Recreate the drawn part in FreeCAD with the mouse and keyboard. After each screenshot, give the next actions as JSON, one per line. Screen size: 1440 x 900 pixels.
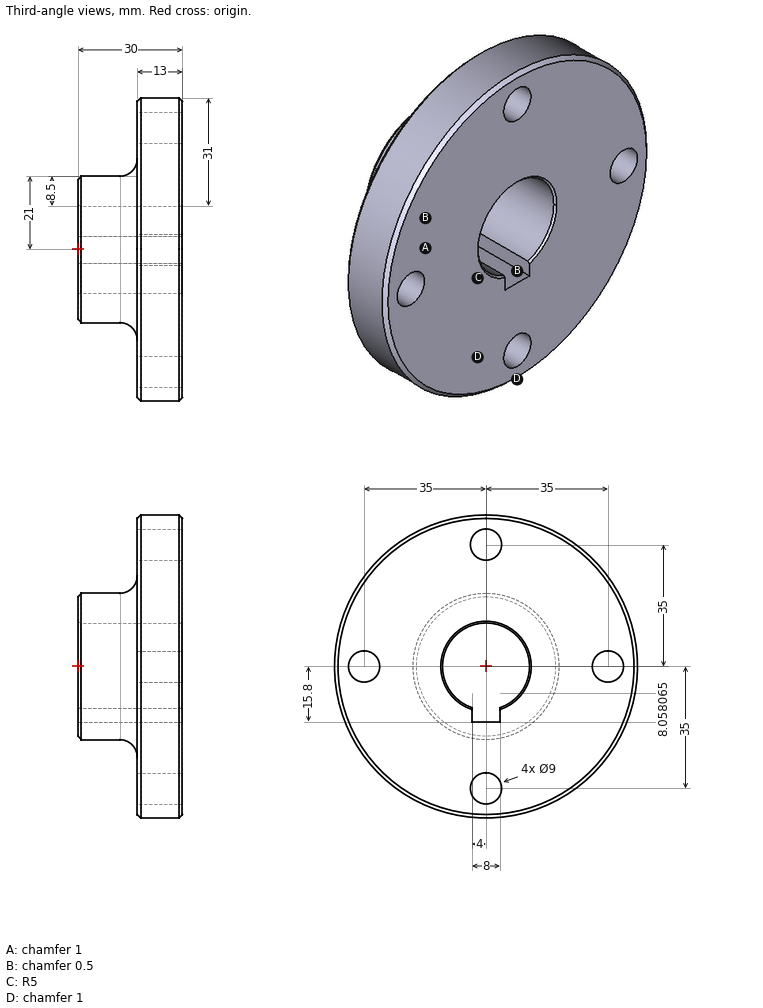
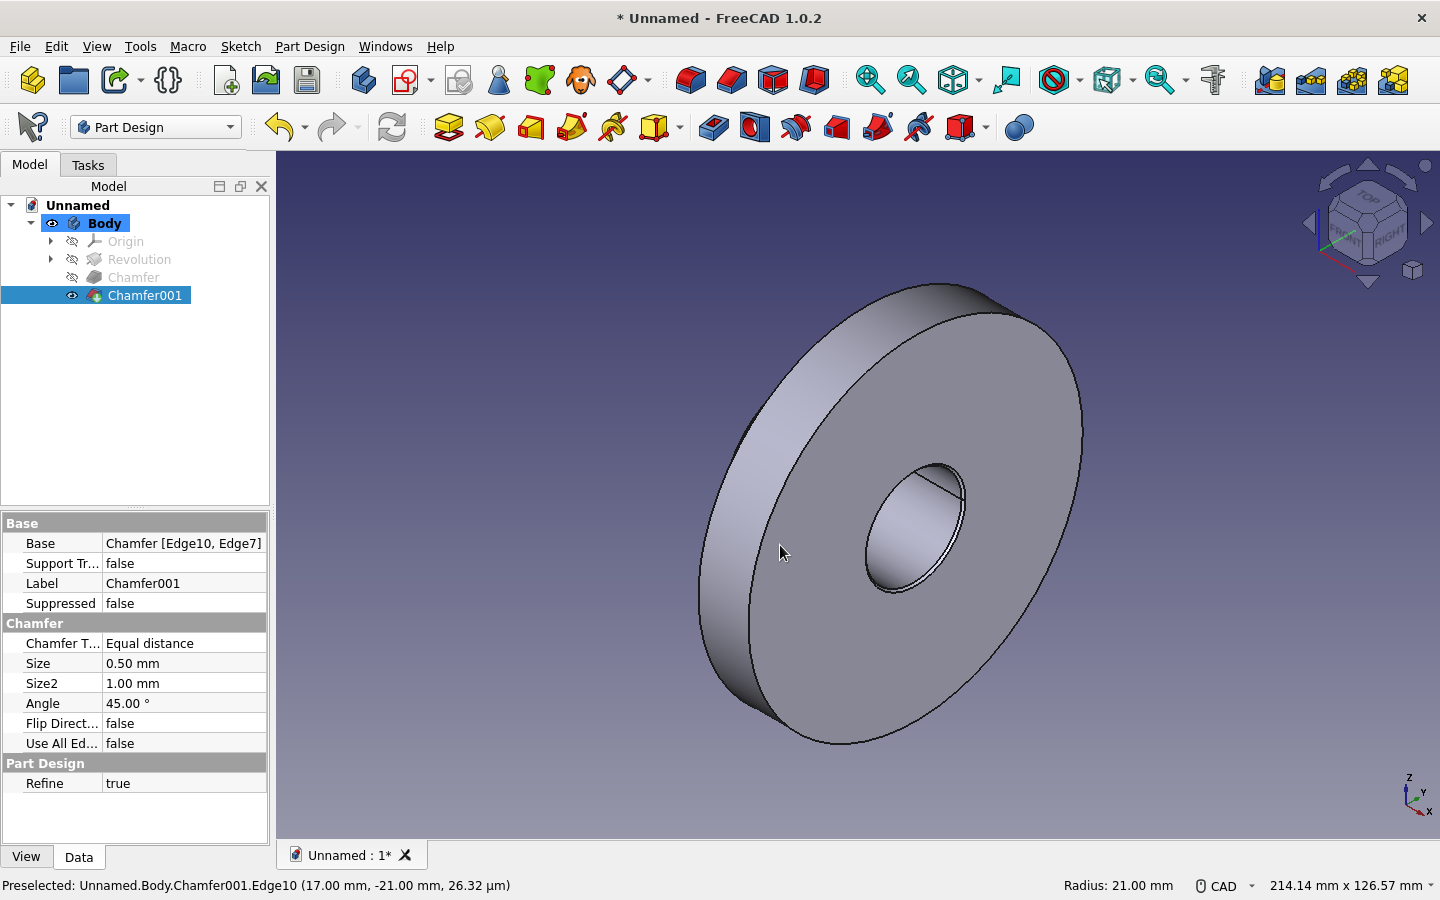
{"action": "left_click", "coordinate": [691, 80]}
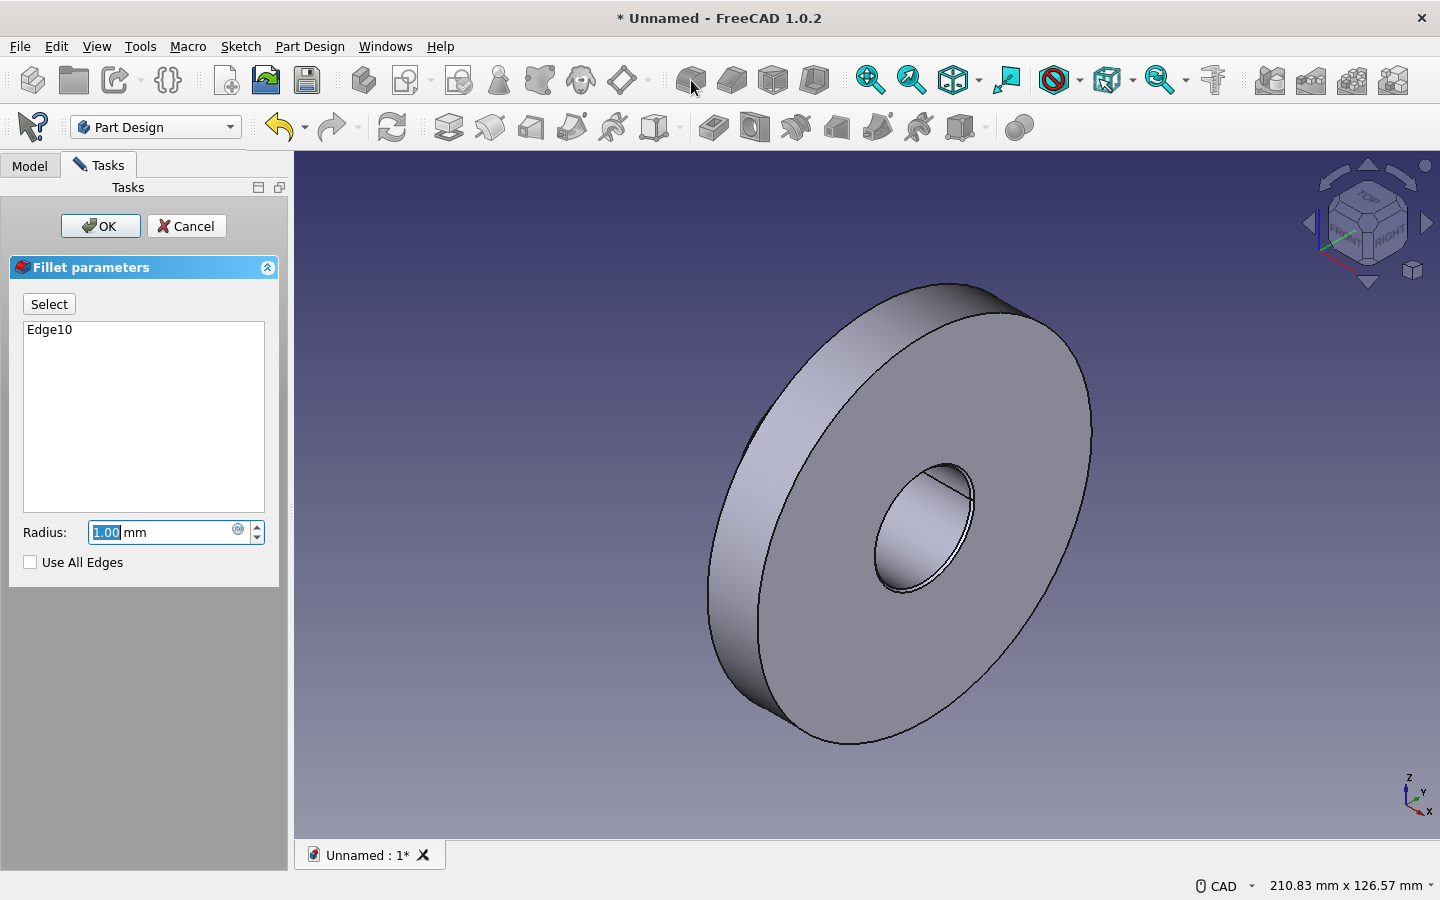
{"action": "type", "text": "5"}
{"action": "key", "text": "Tab"}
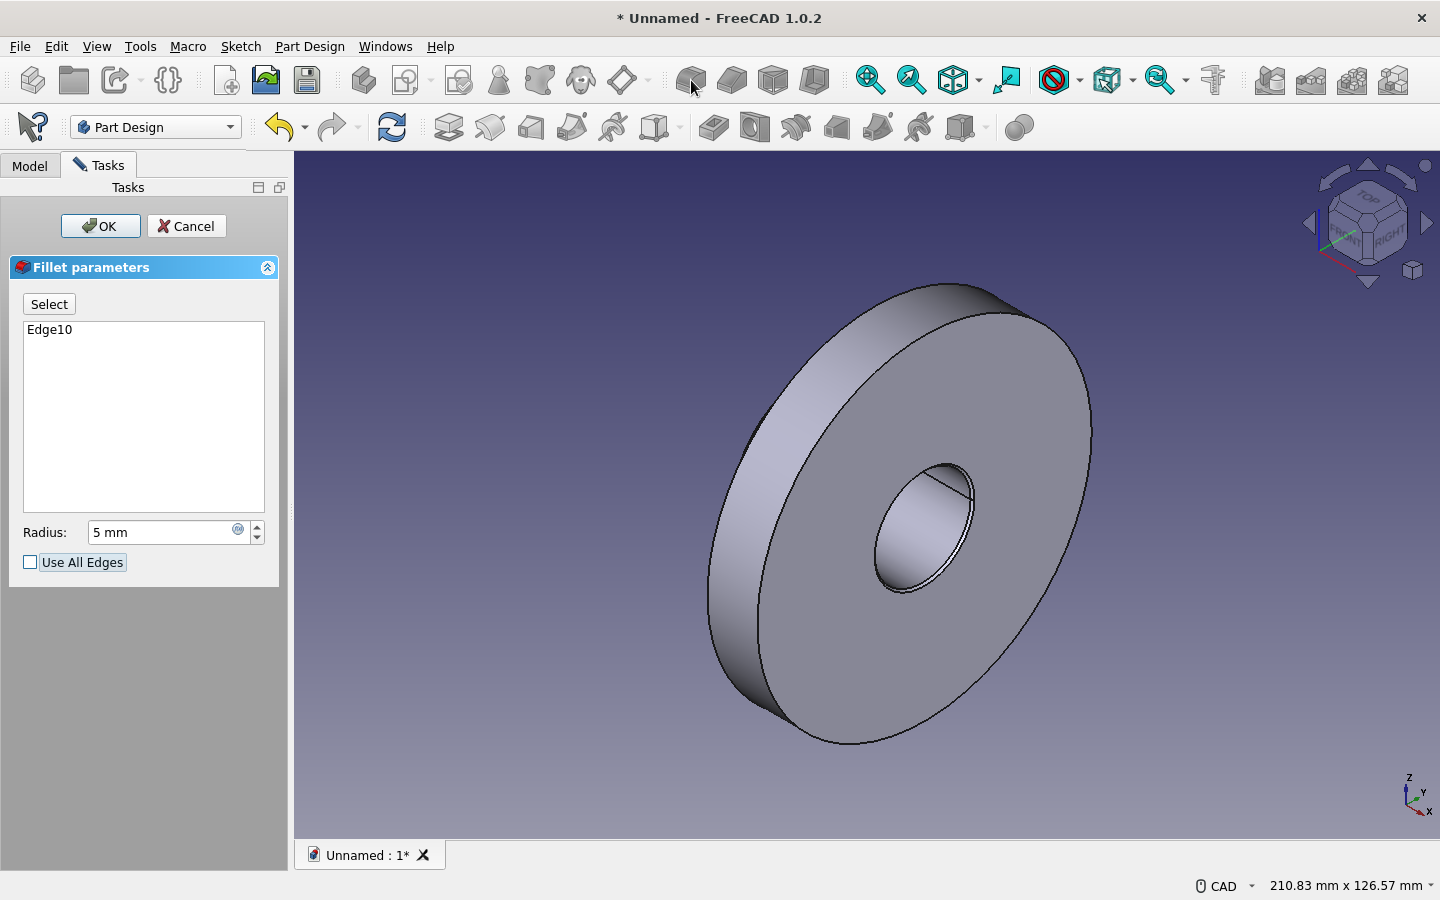
{"action": "left_click", "coordinate": [101, 226]}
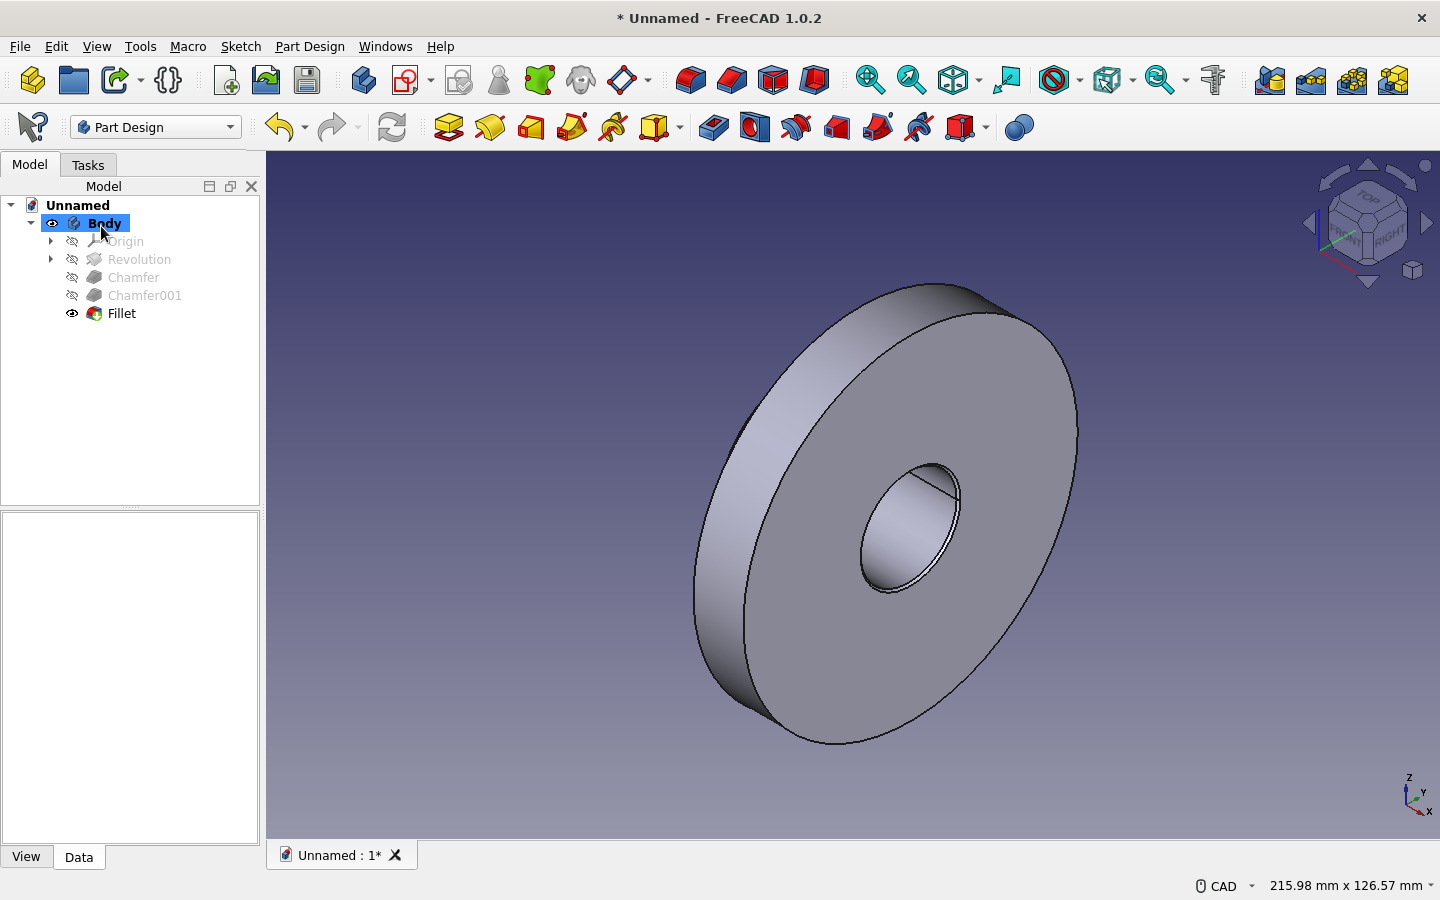
{"action": "left_click", "coordinate": [743, 624]}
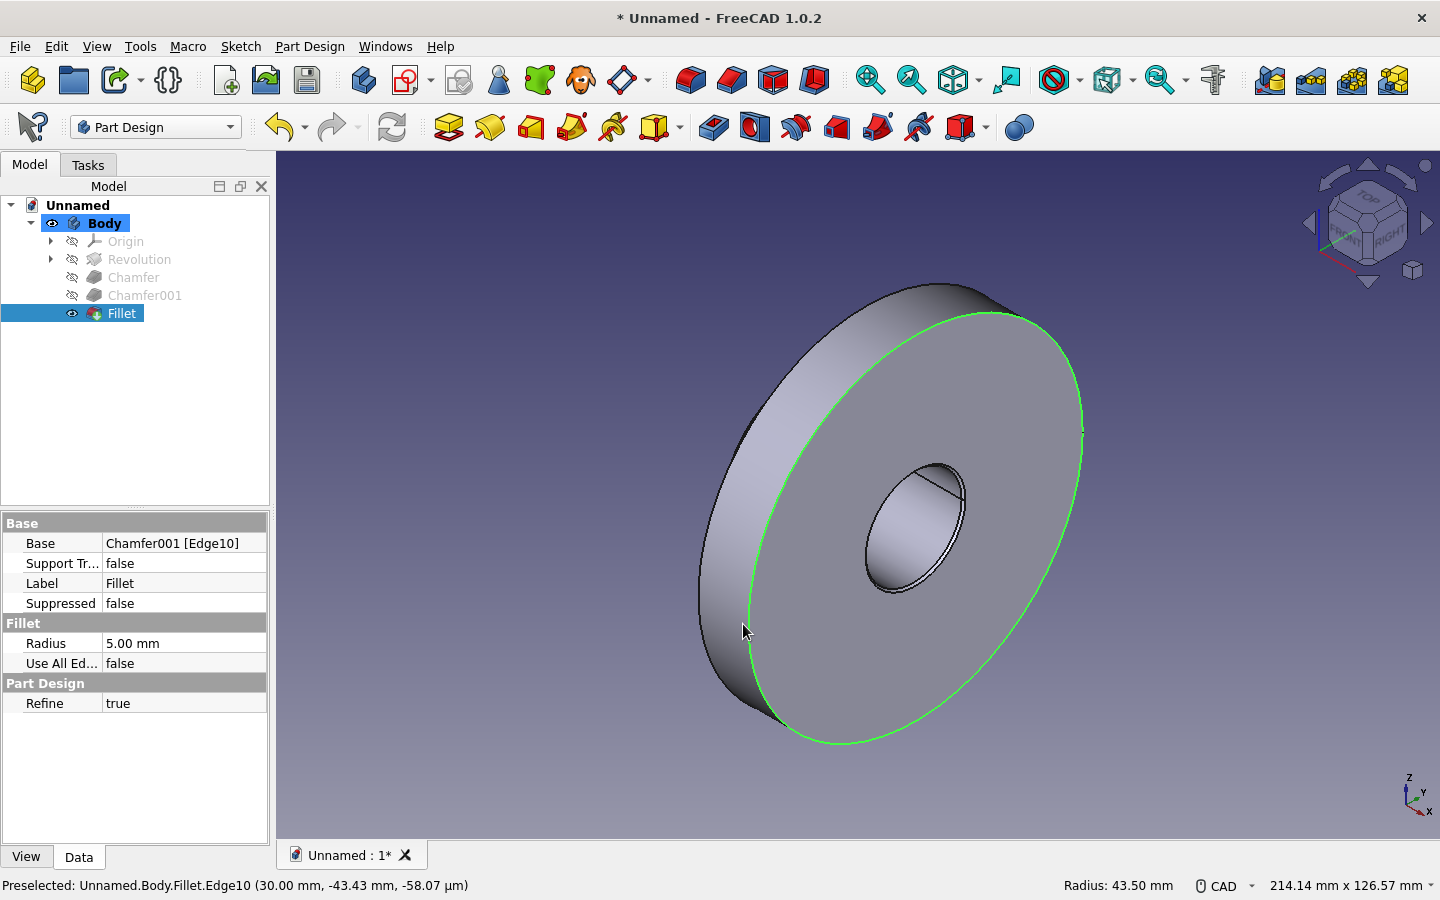
{"action": "key", "text": "2"}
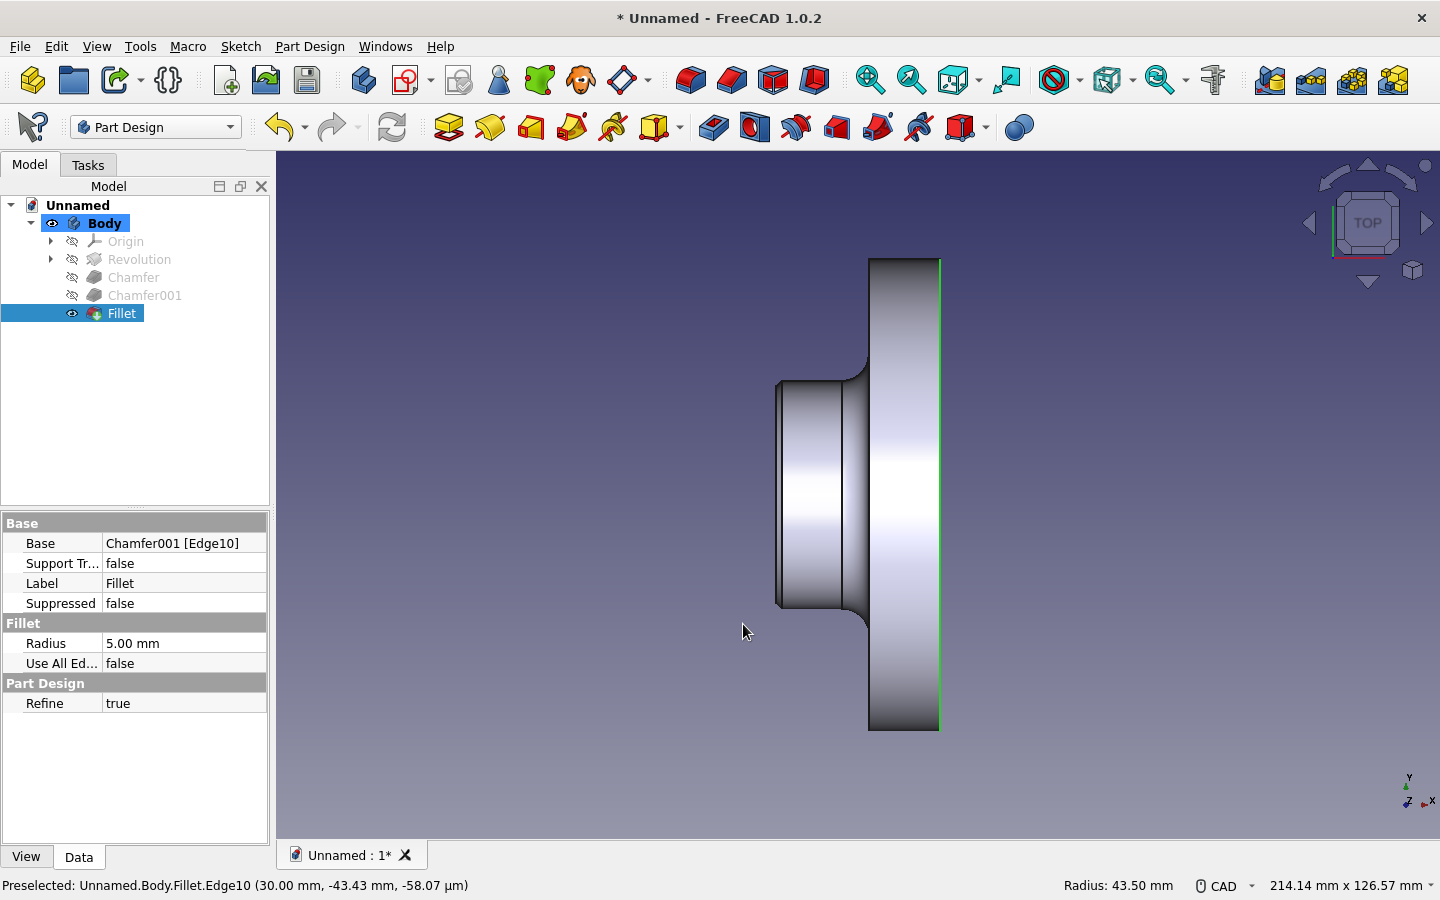
{"action": "left_click", "coordinate": [869, 685], "text": "ctrl"}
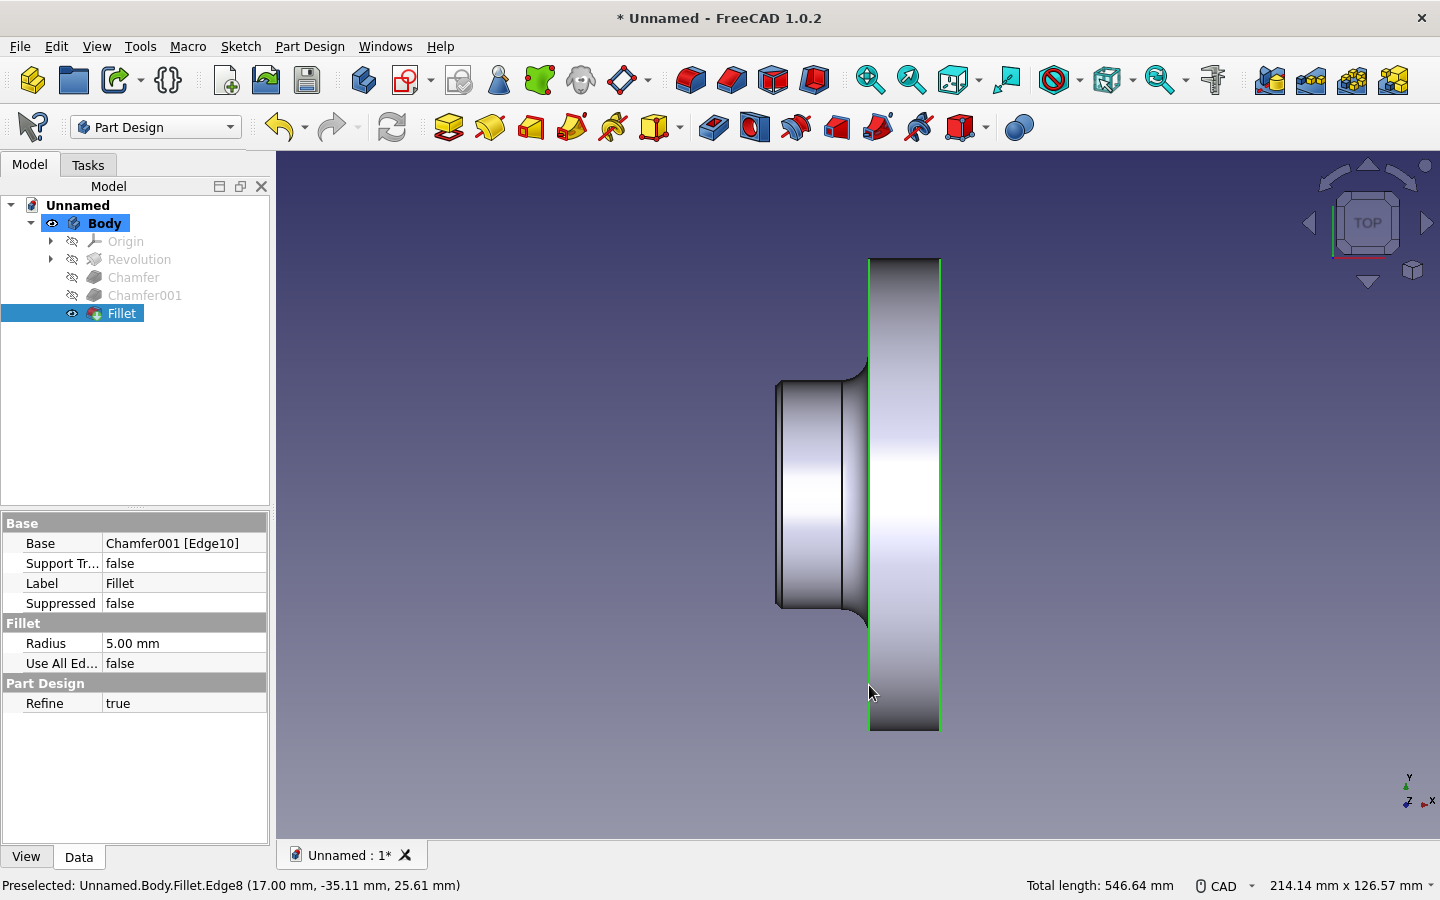
{"action": "left_click", "coordinate": [732, 80]}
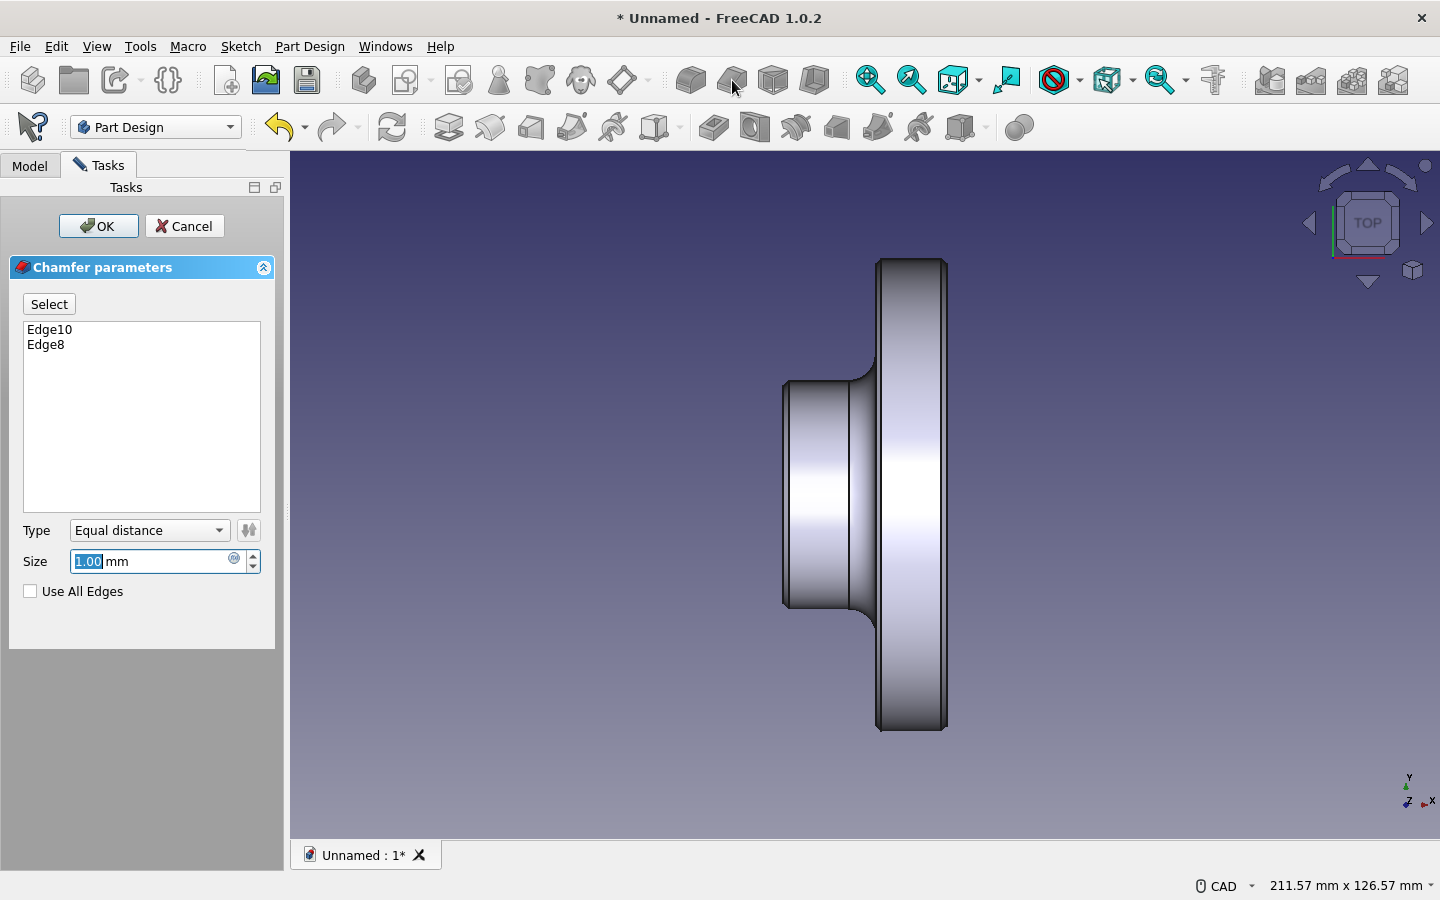
{"action": "type", "text": "1"}
{"action": "key", "text": "Tab"}